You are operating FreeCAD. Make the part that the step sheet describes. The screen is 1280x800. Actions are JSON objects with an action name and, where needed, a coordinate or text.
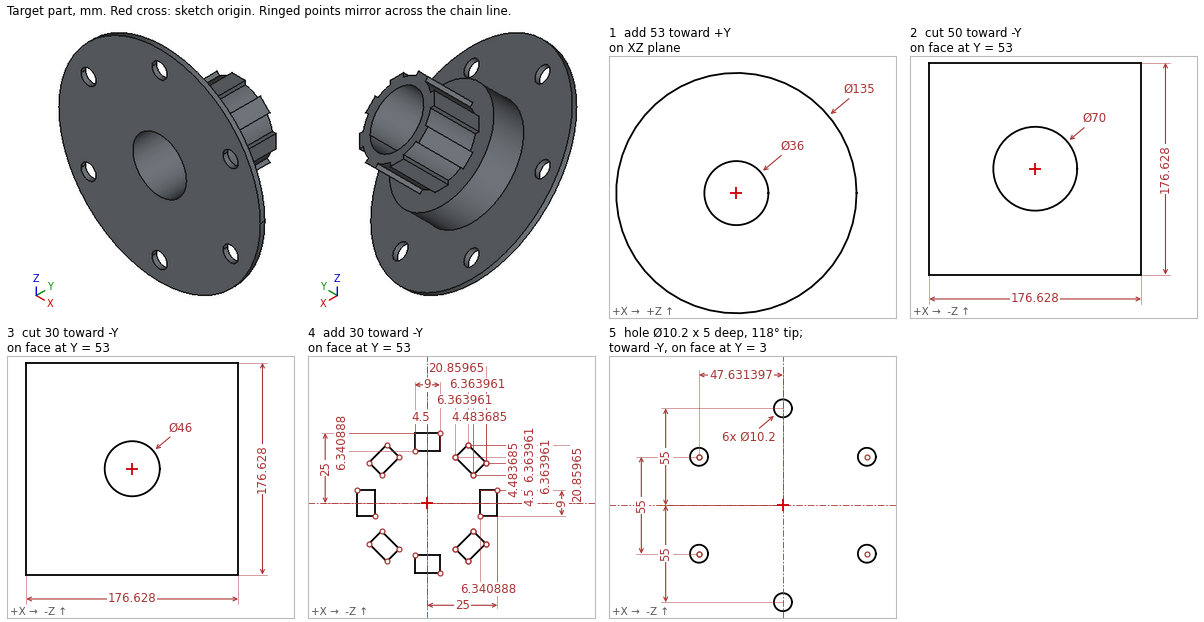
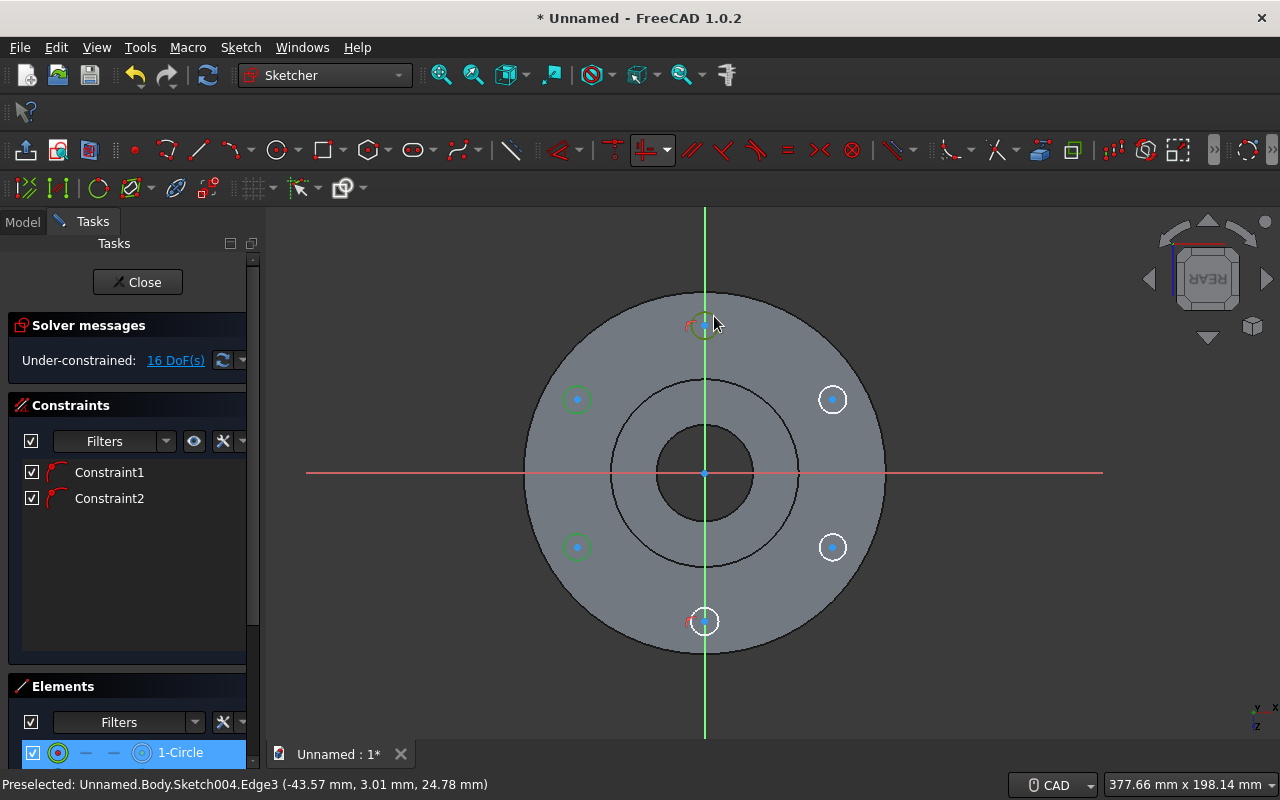
{"action": "scroll", "coordinate": [714, 612], "scroll_direction": "up", "scroll_amount": 2}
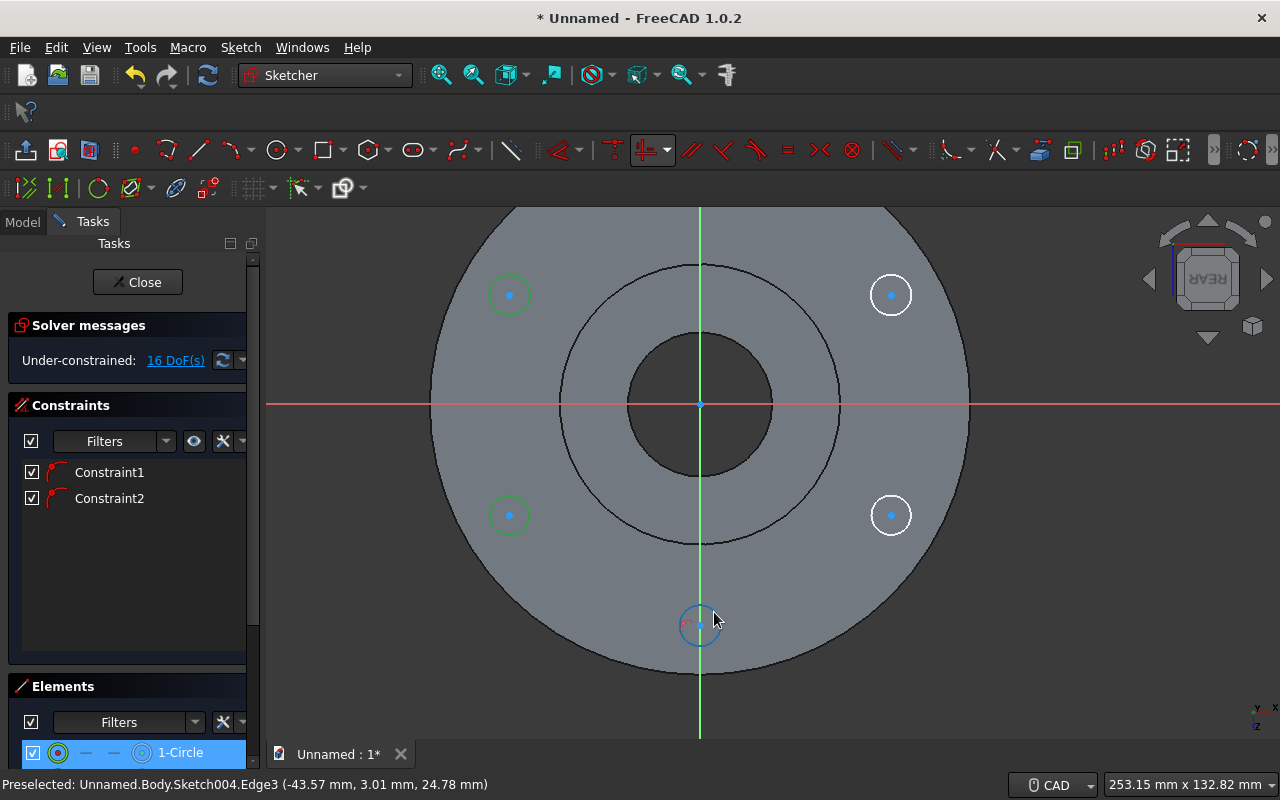
{"action": "left_click", "coordinate": [715, 611]}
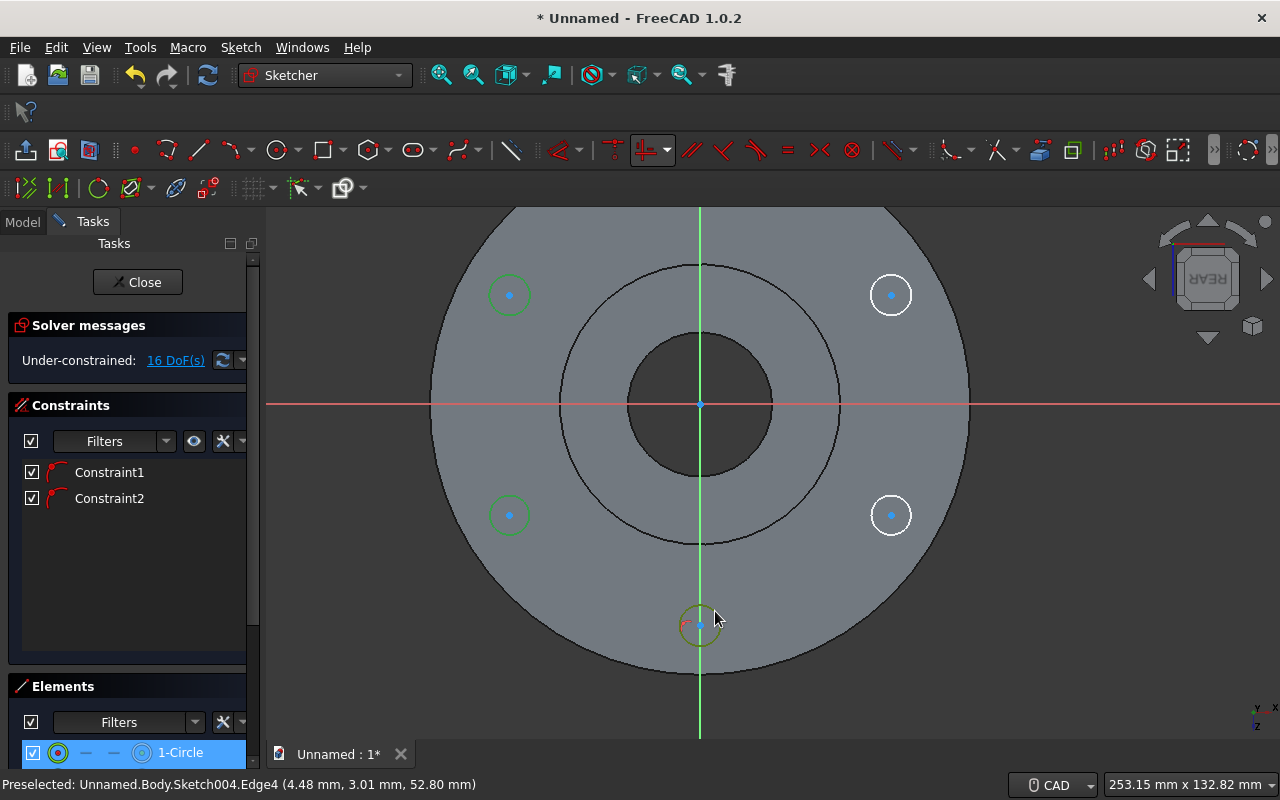
{"action": "left_click", "coordinate": [905, 501]}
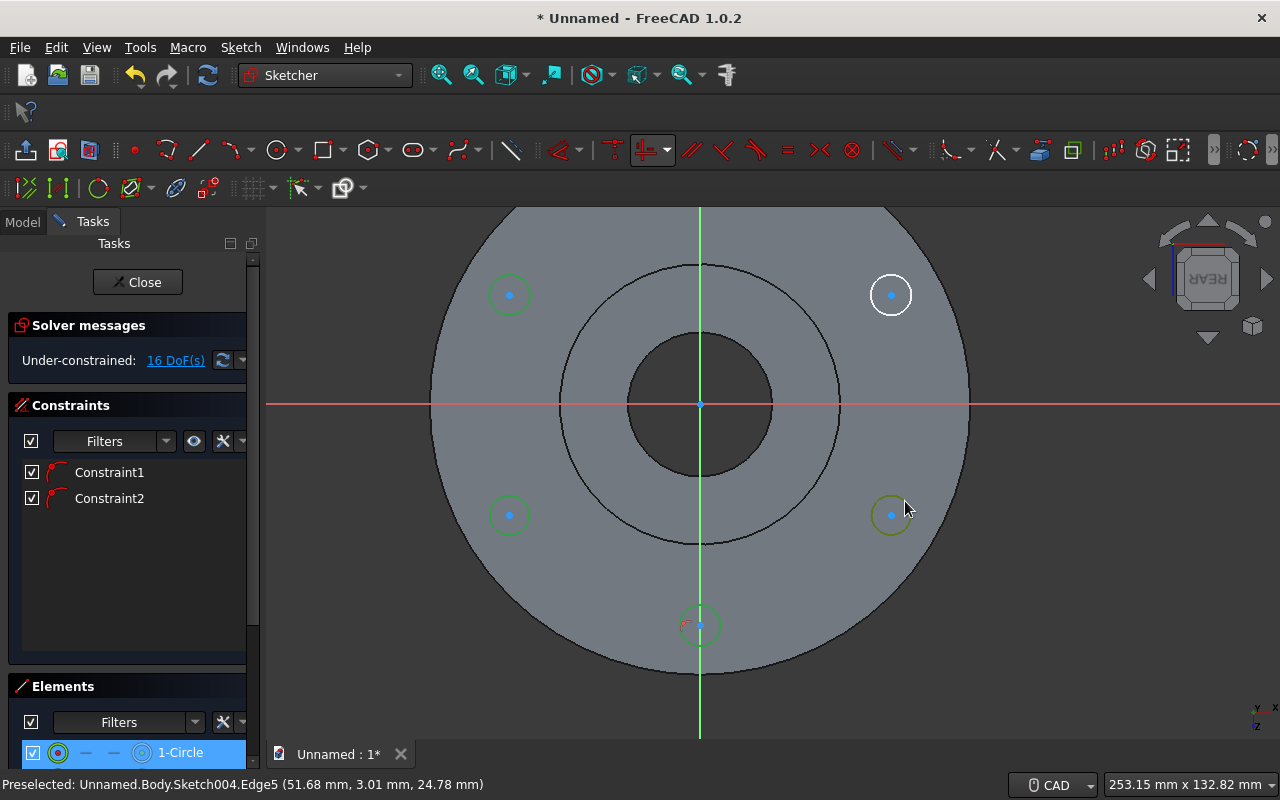
{"action": "left_click", "coordinate": [905, 281]}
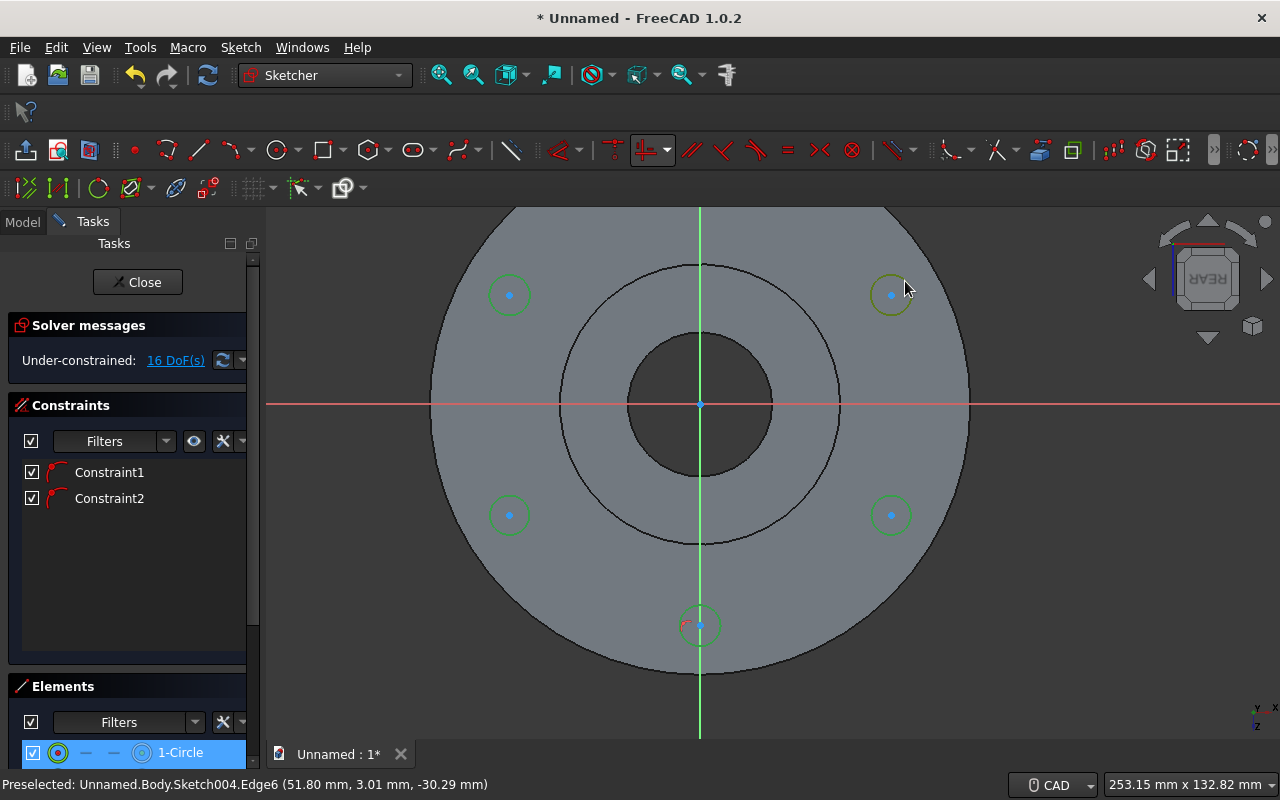
{"action": "left_click", "coordinate": [788, 150]}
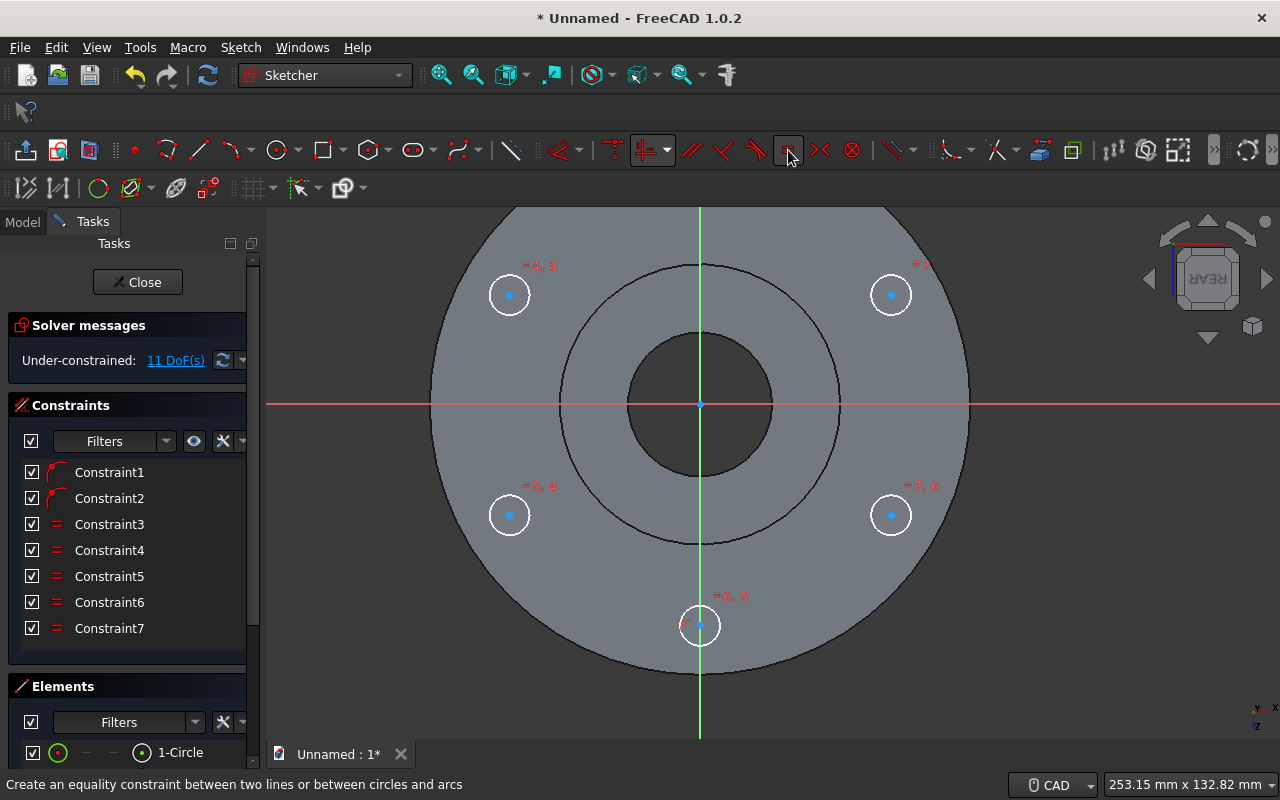
{"action": "left_click", "coordinate": [510, 295]}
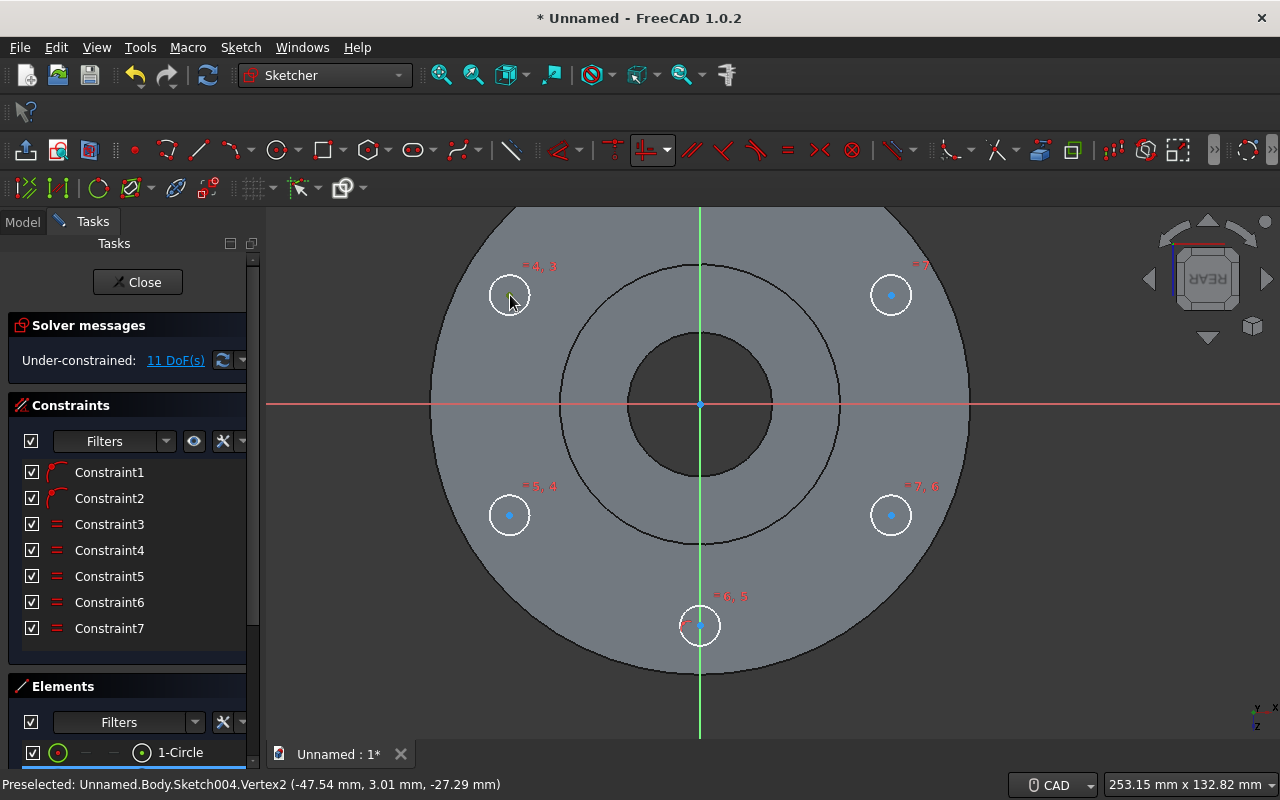
{"action": "left_click", "coordinate": [510, 515]}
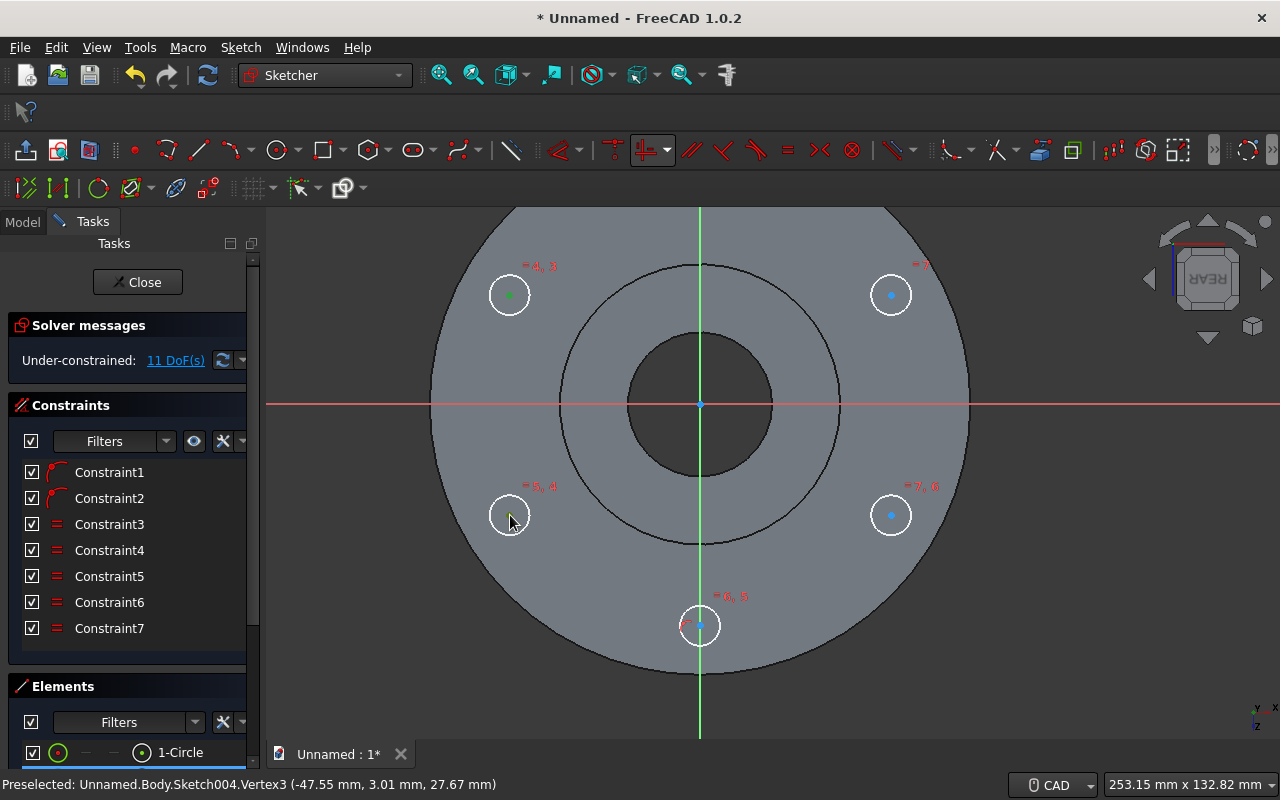
{"action": "left_click", "coordinate": [353, 404]}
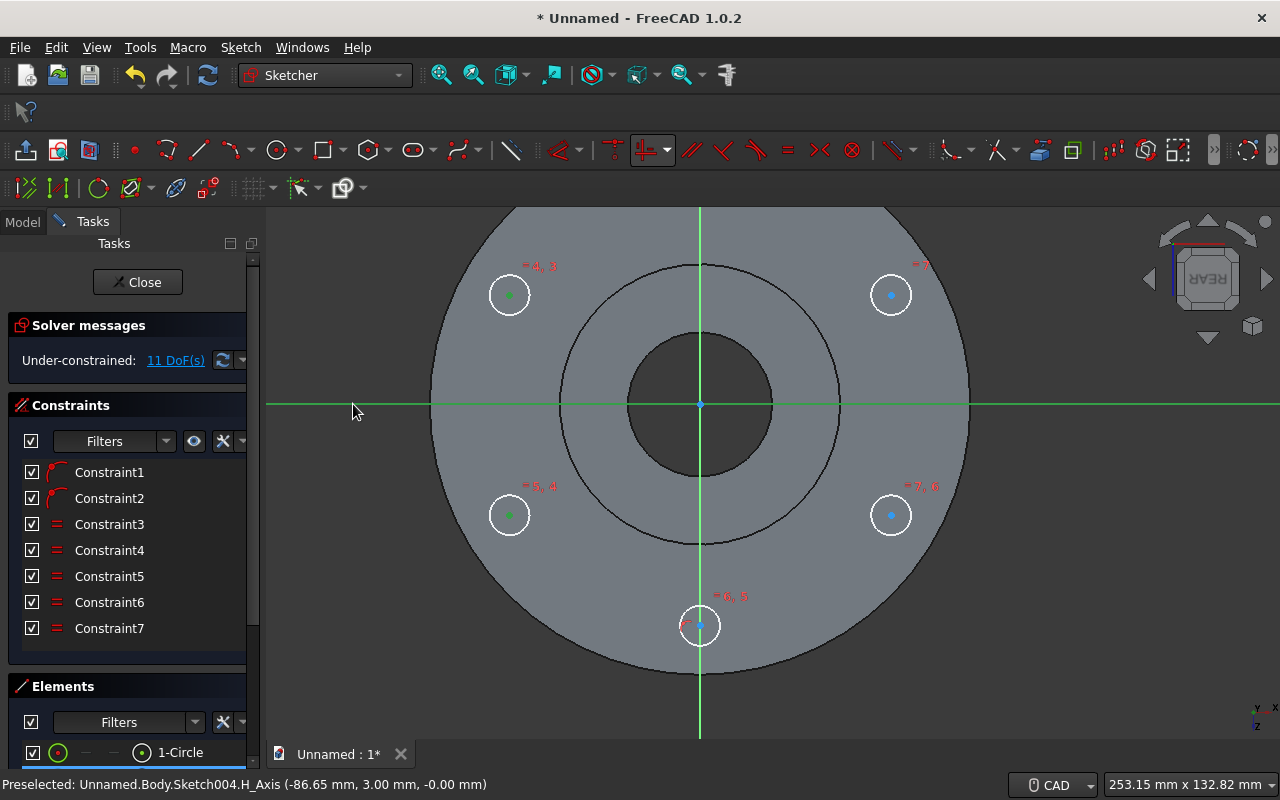
{"action": "left_click", "coordinate": [820, 150]}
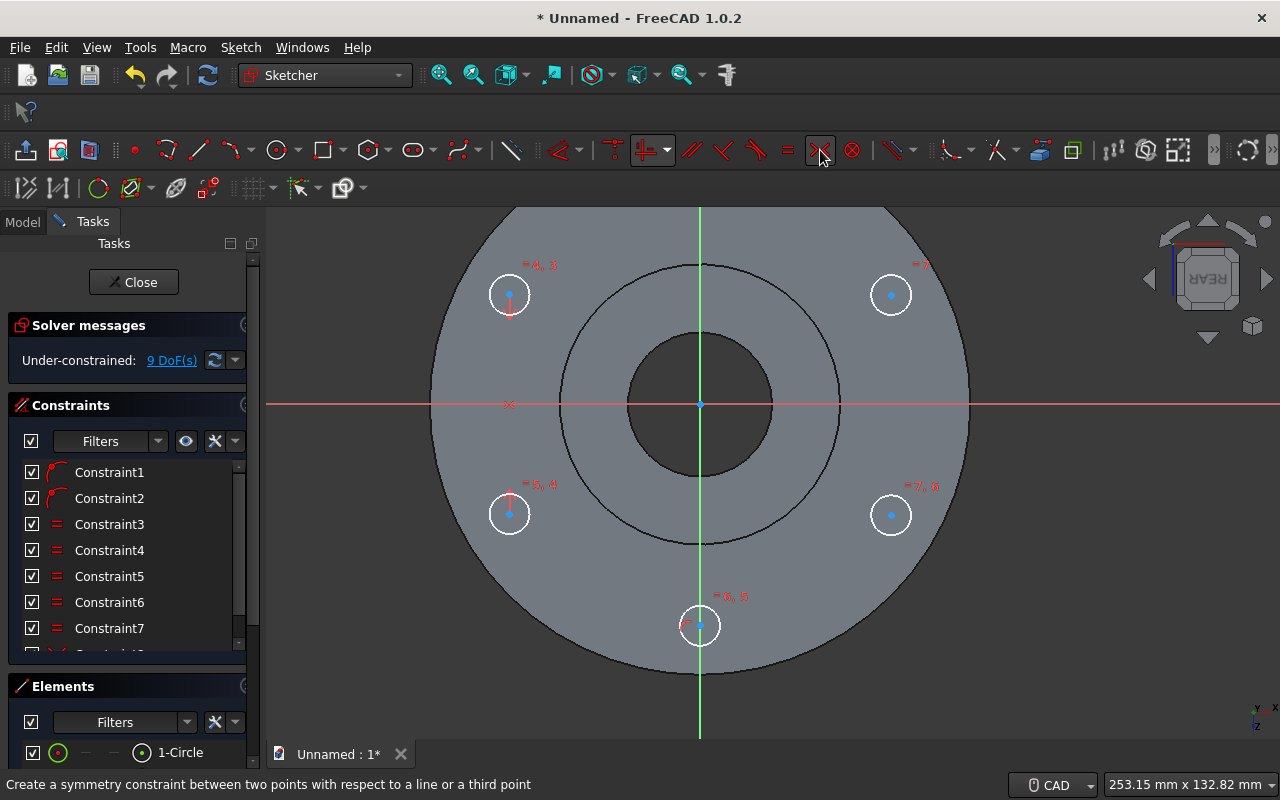
{"action": "left_click", "coordinate": [510, 514]}